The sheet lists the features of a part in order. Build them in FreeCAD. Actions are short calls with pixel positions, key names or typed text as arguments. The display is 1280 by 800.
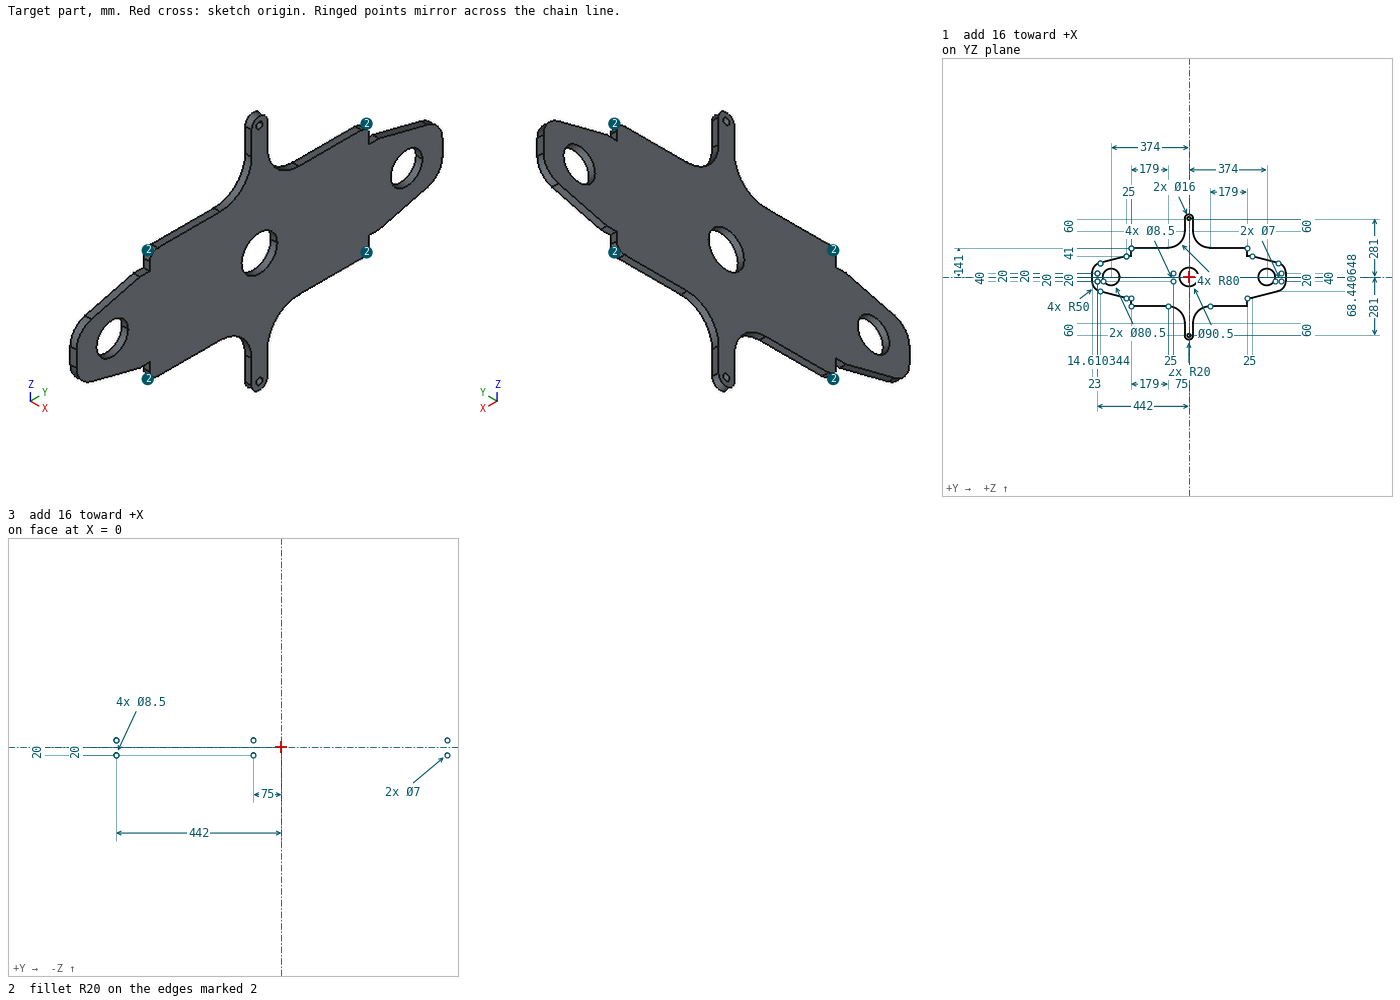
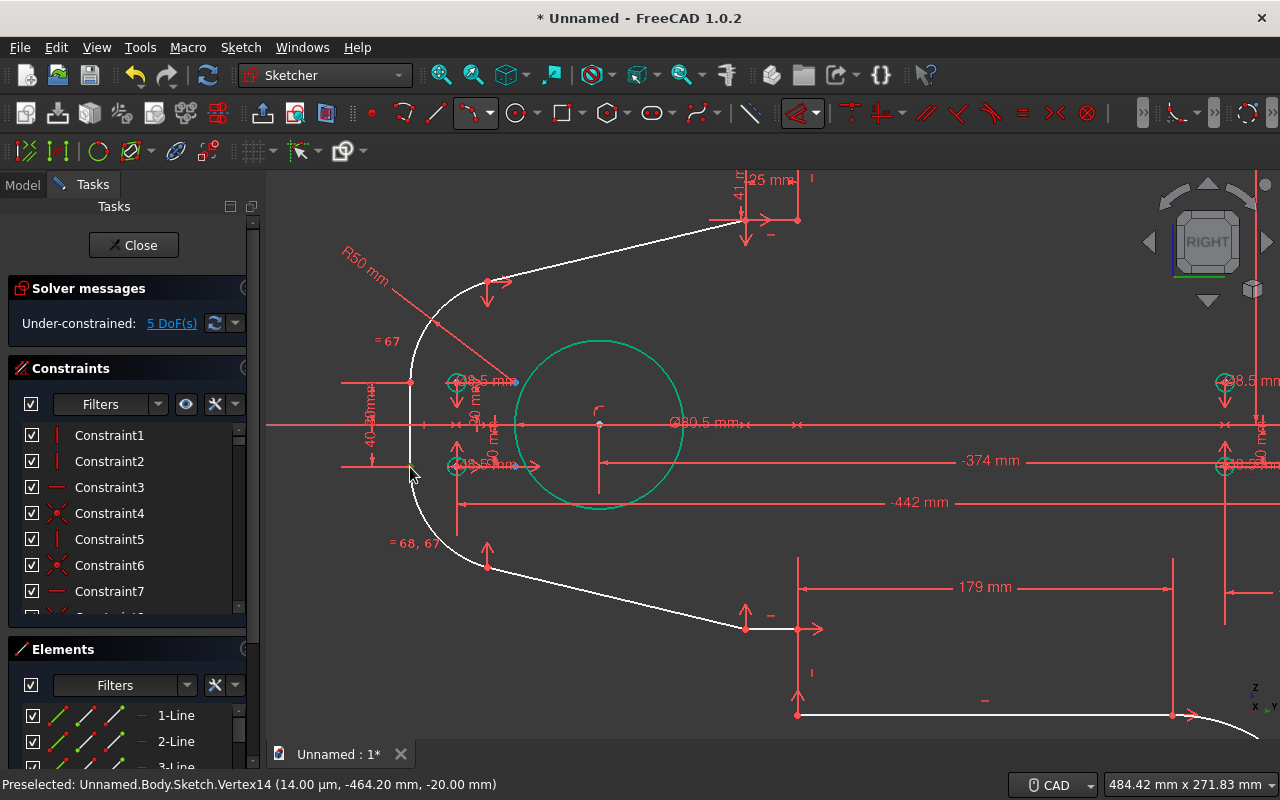
click(457, 467)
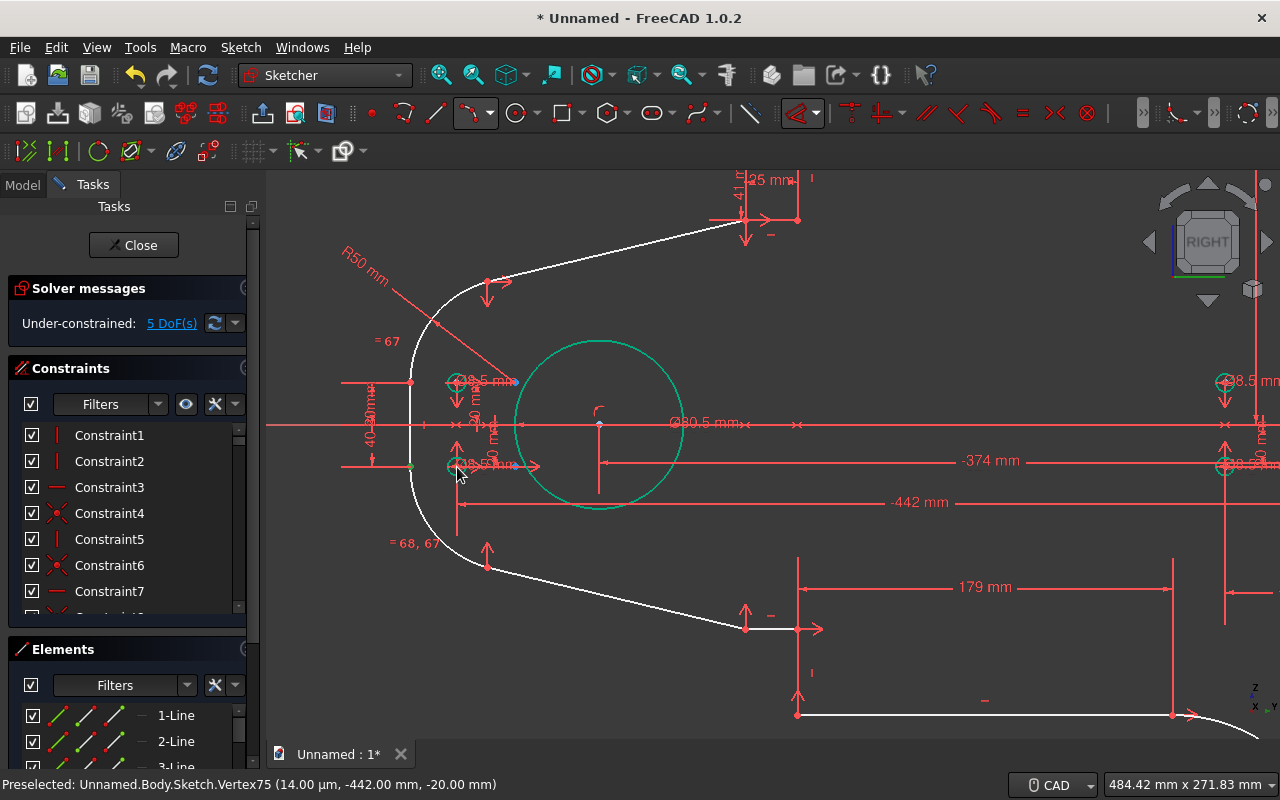
key(l)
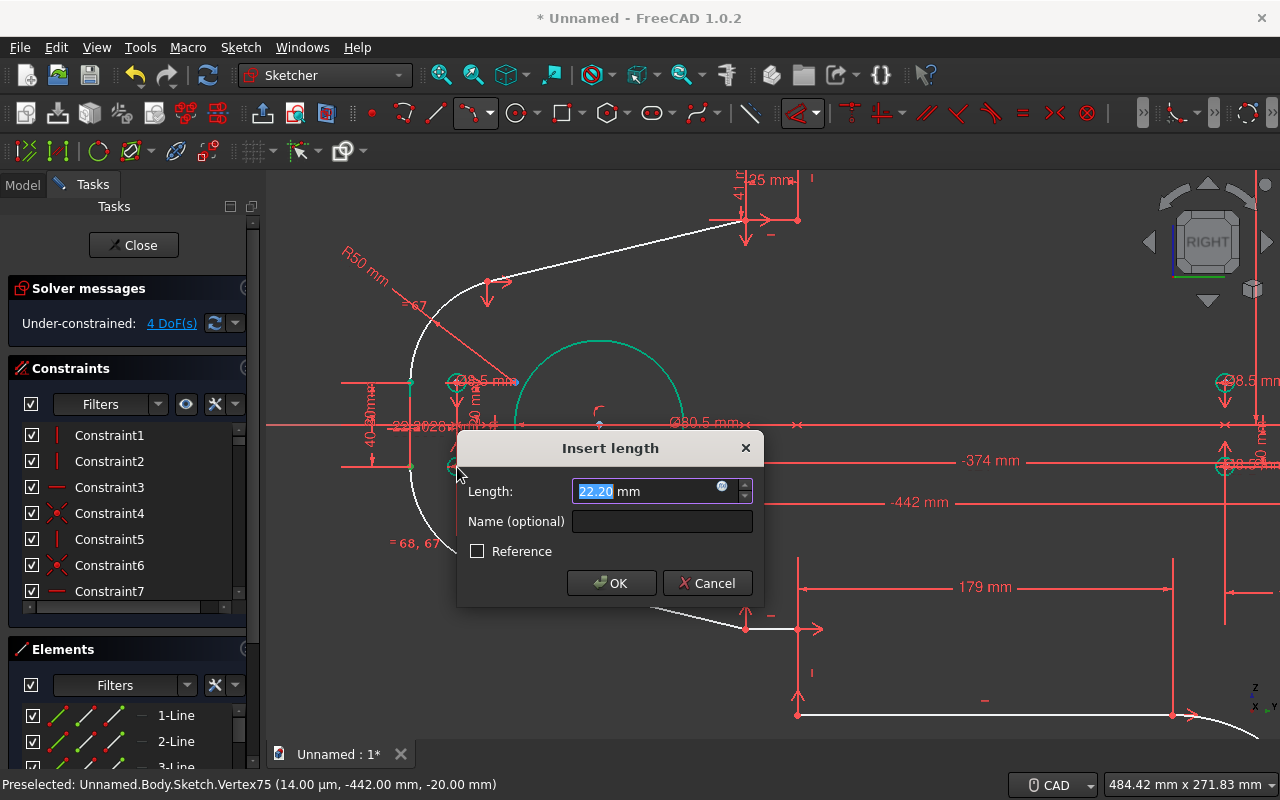
text(23)
key(Return)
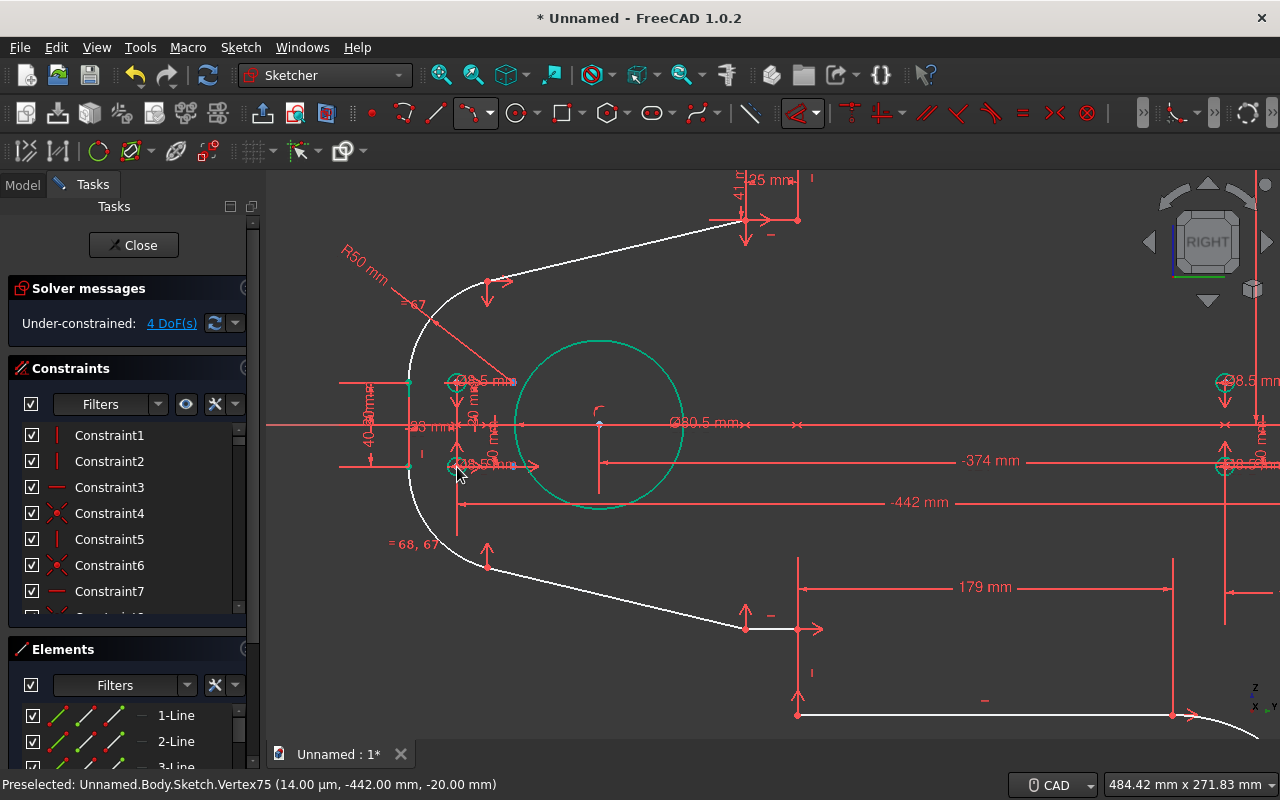
scroll(412, 467, down, 6)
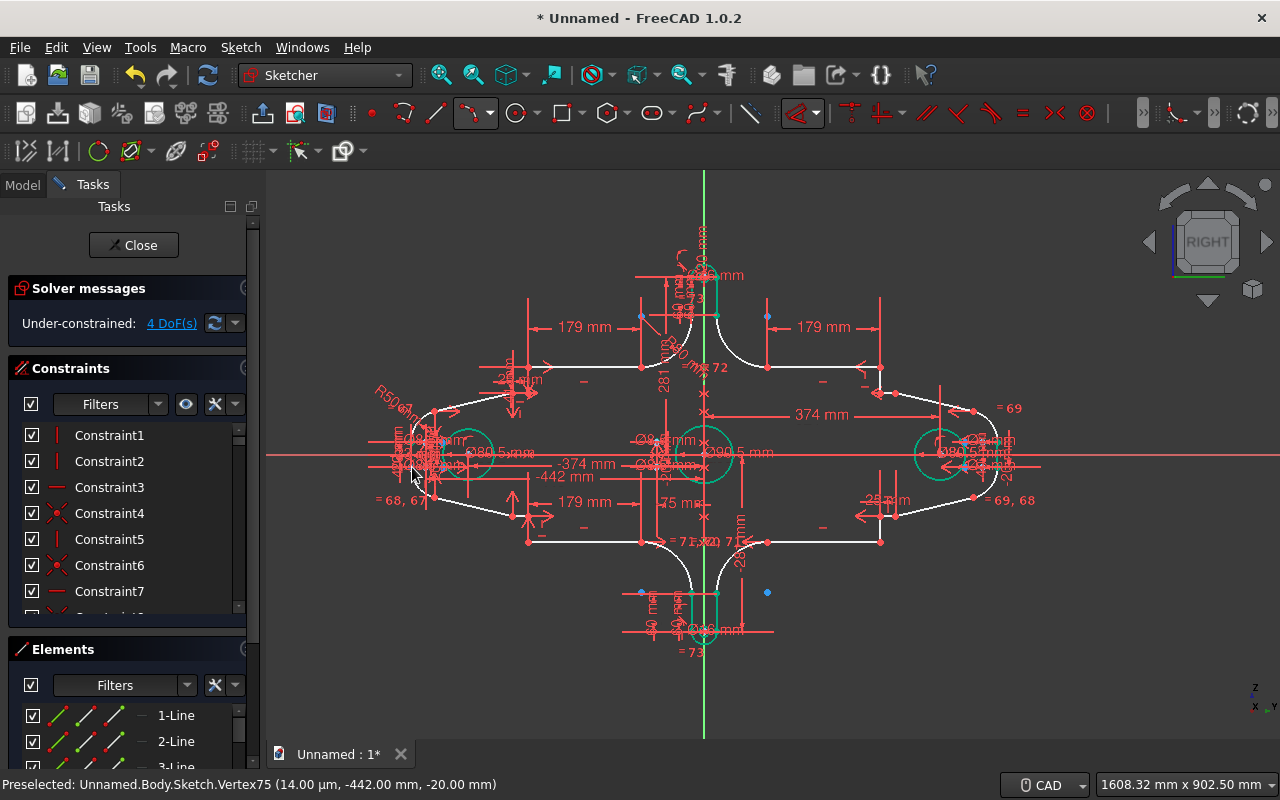
scroll(641, 542, up, 5)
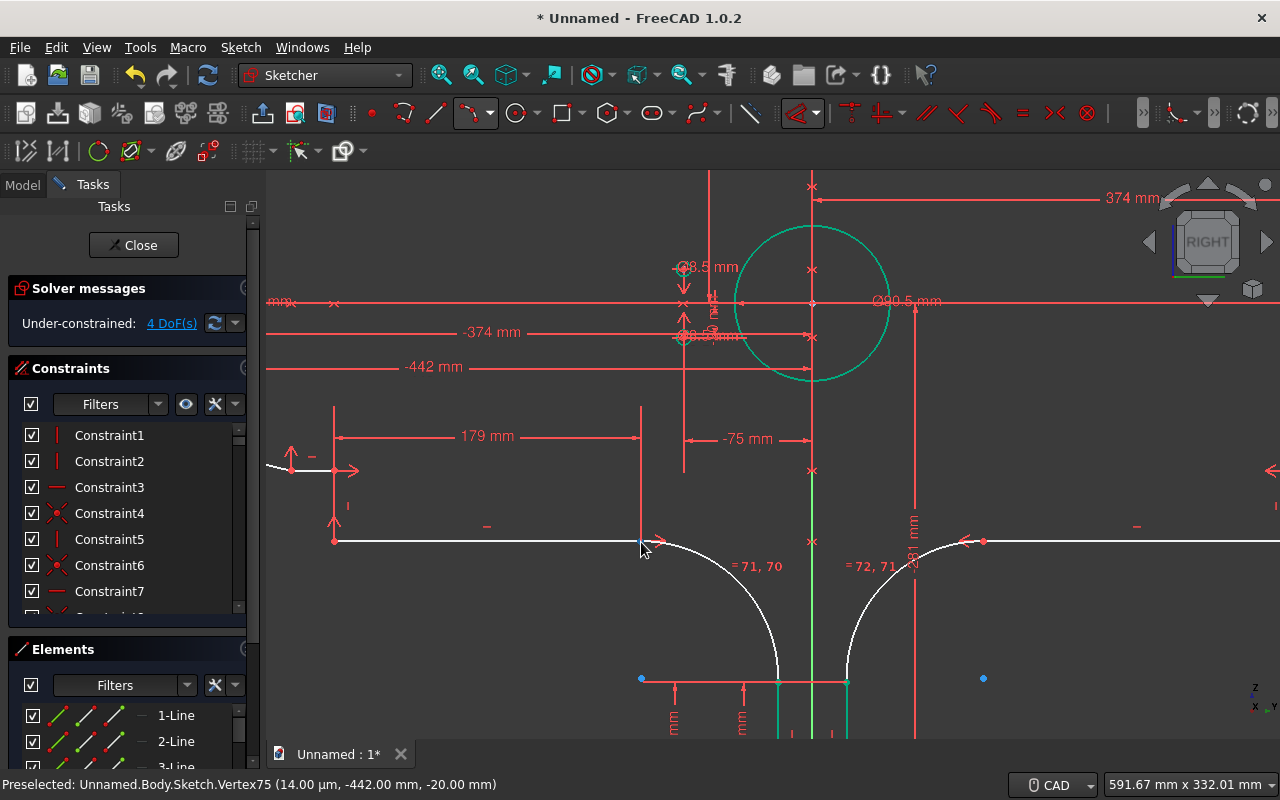
click(641, 541)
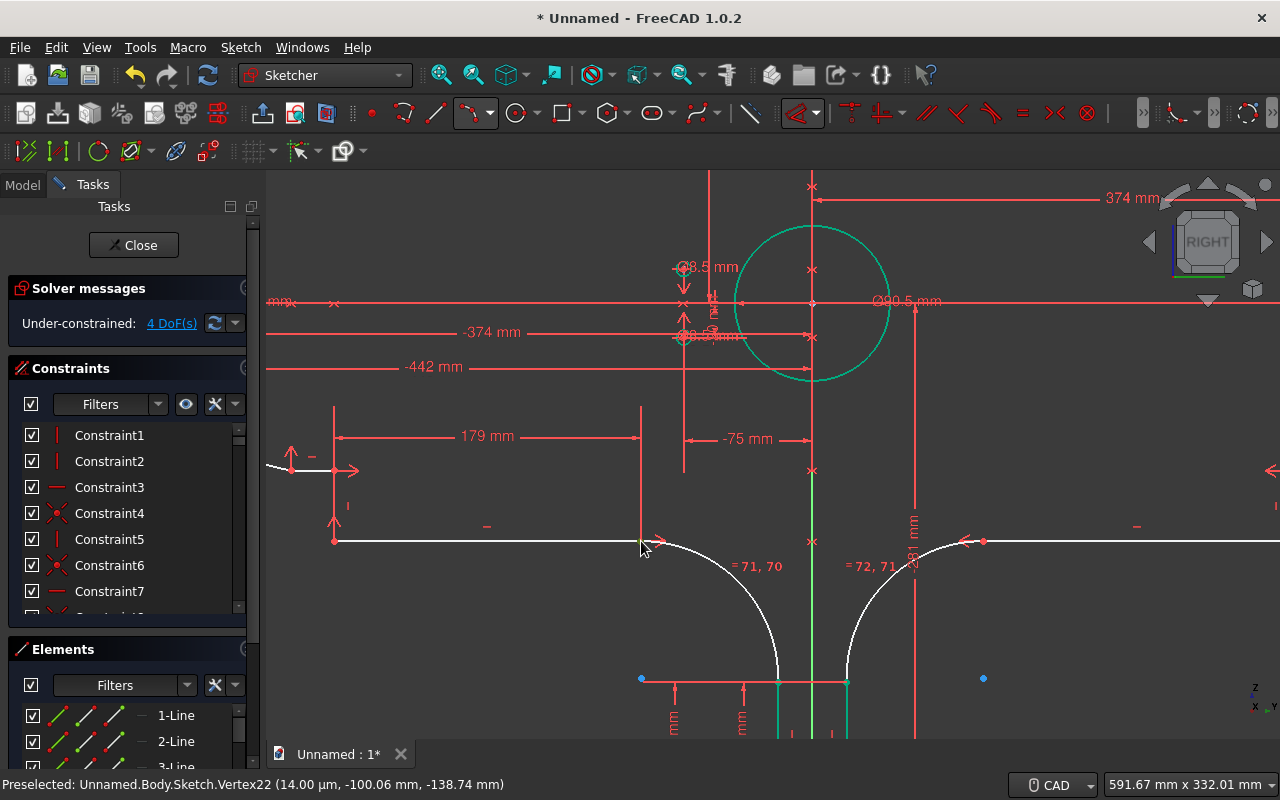
click(684, 338)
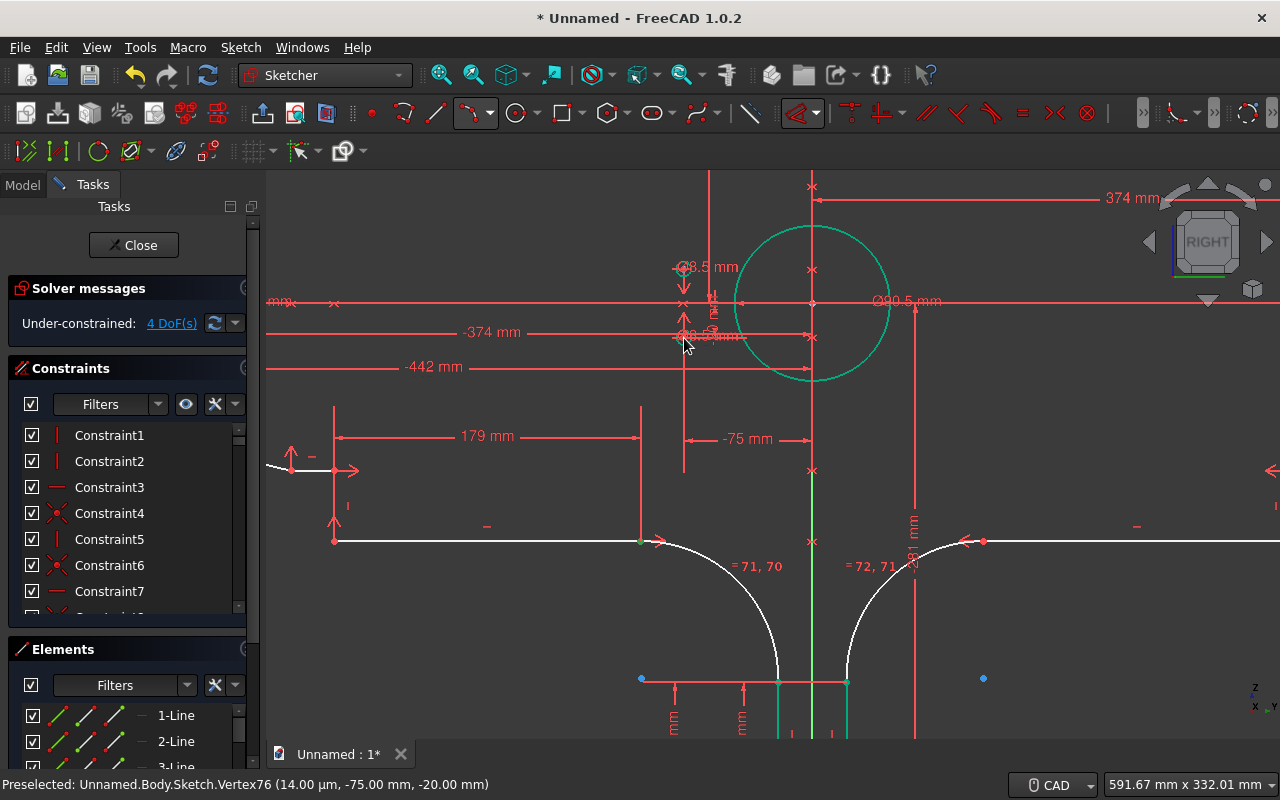
key(l)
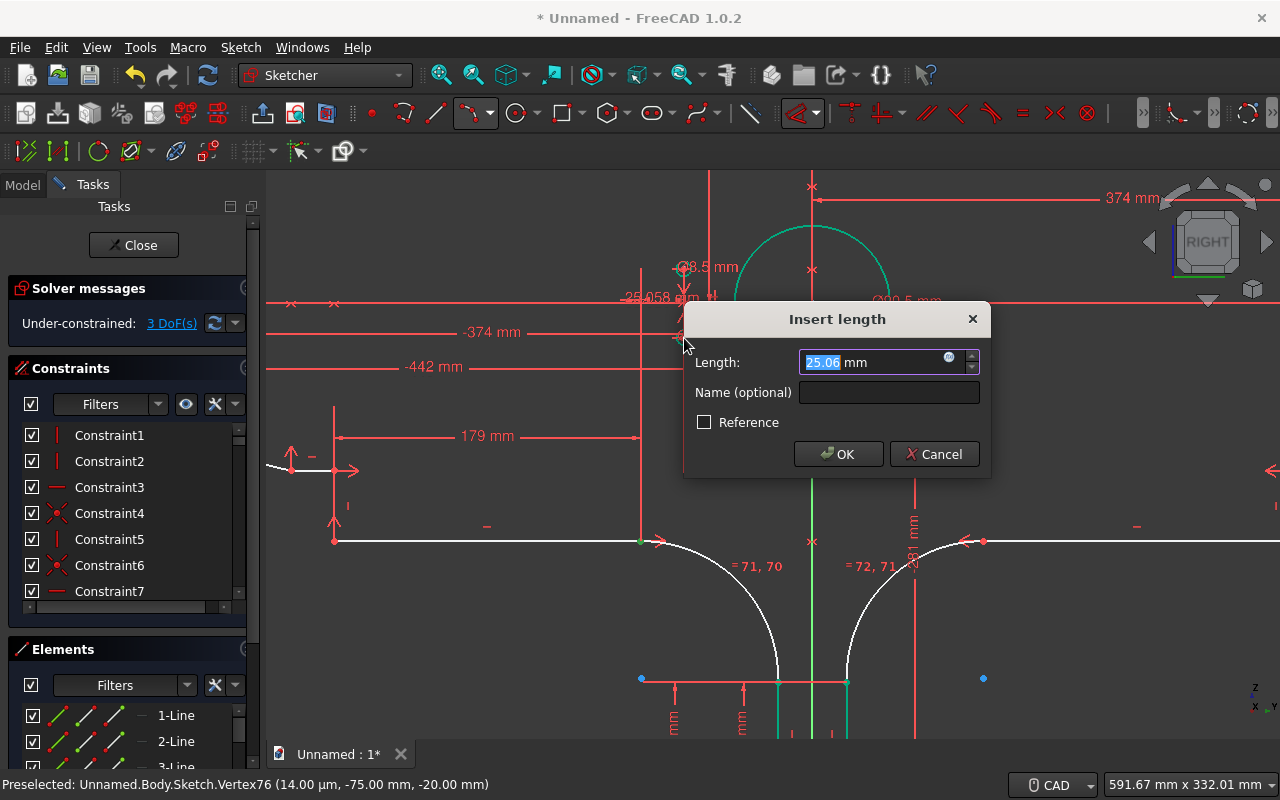
text(25)
key(Return)